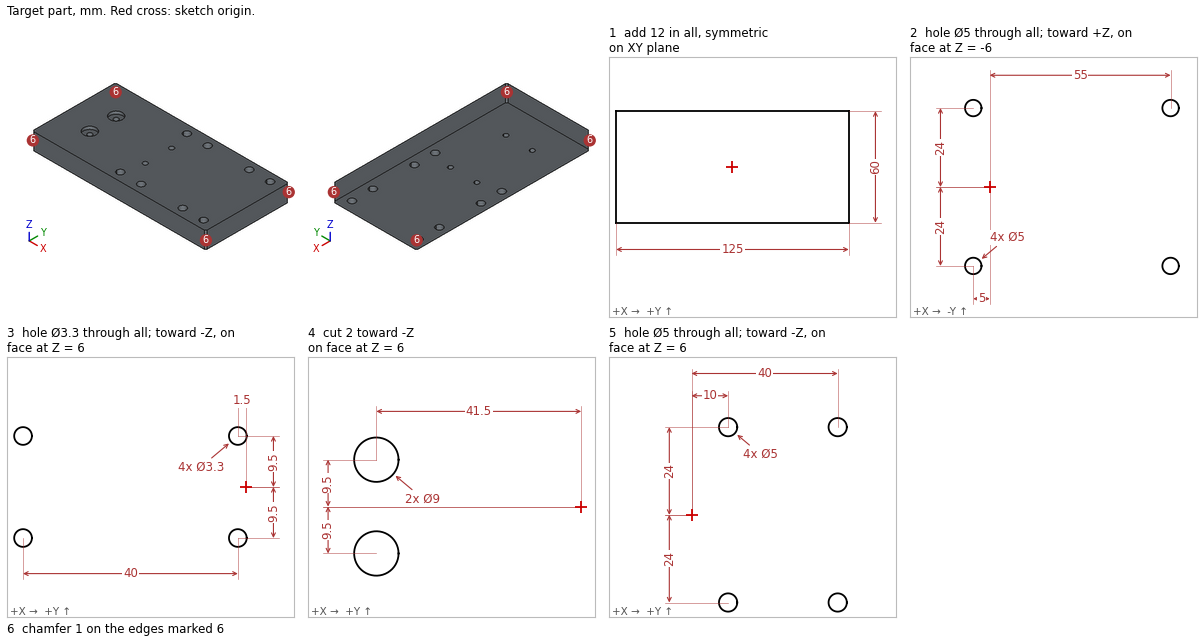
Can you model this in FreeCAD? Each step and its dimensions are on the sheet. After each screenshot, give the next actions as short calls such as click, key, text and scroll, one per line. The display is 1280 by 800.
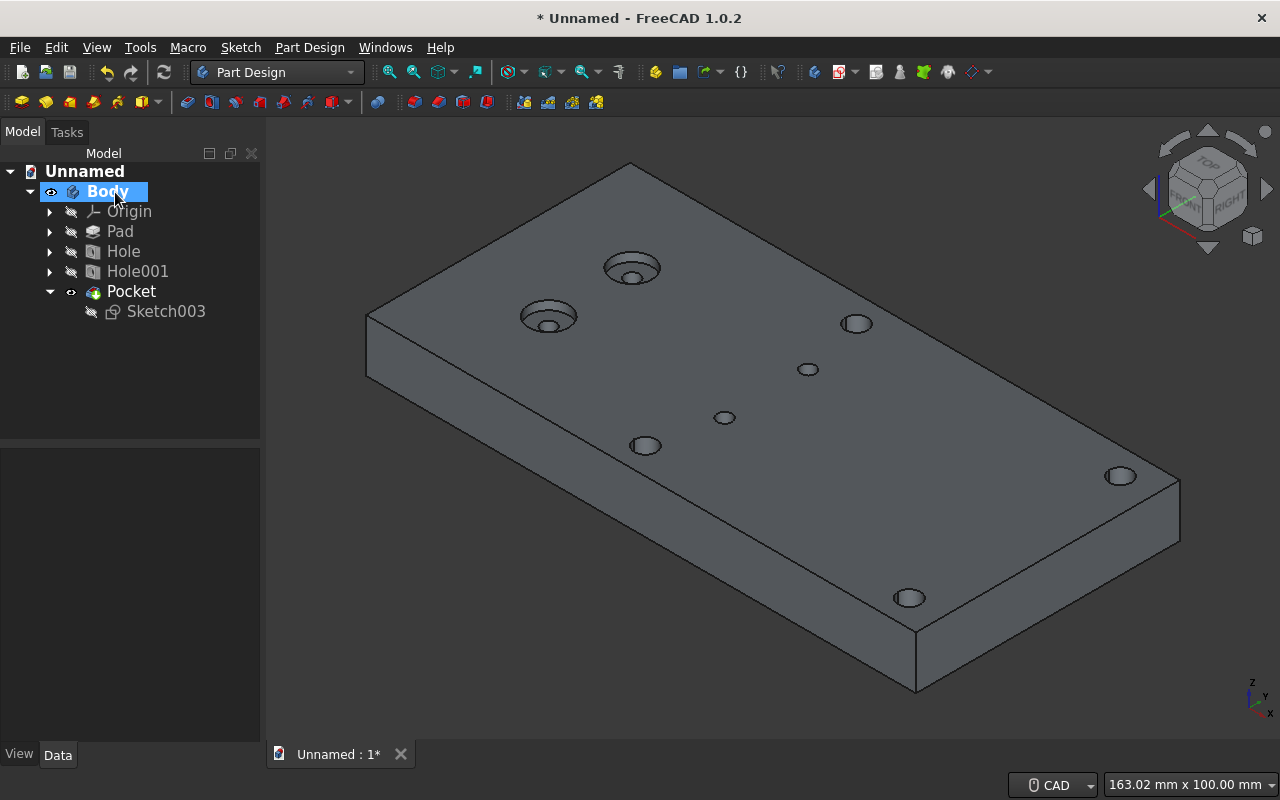
click(930, 487)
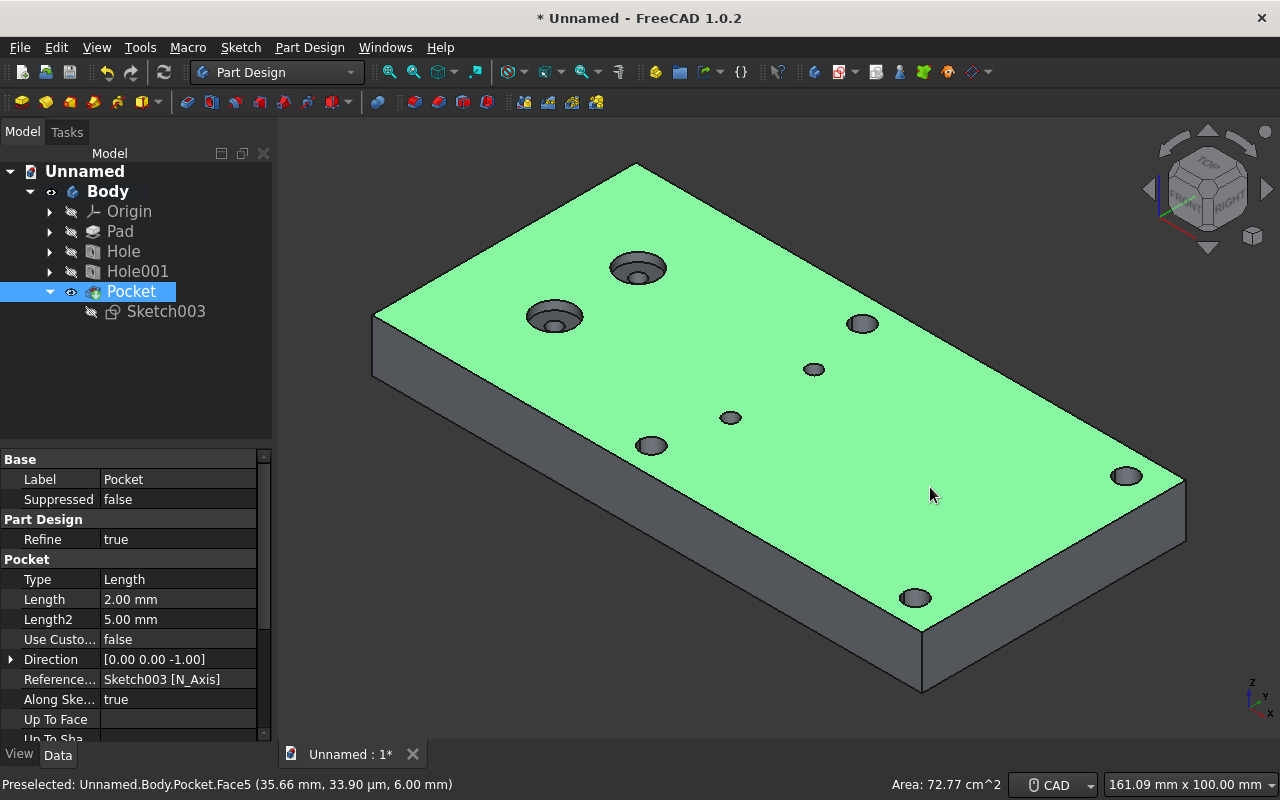
click(840, 72)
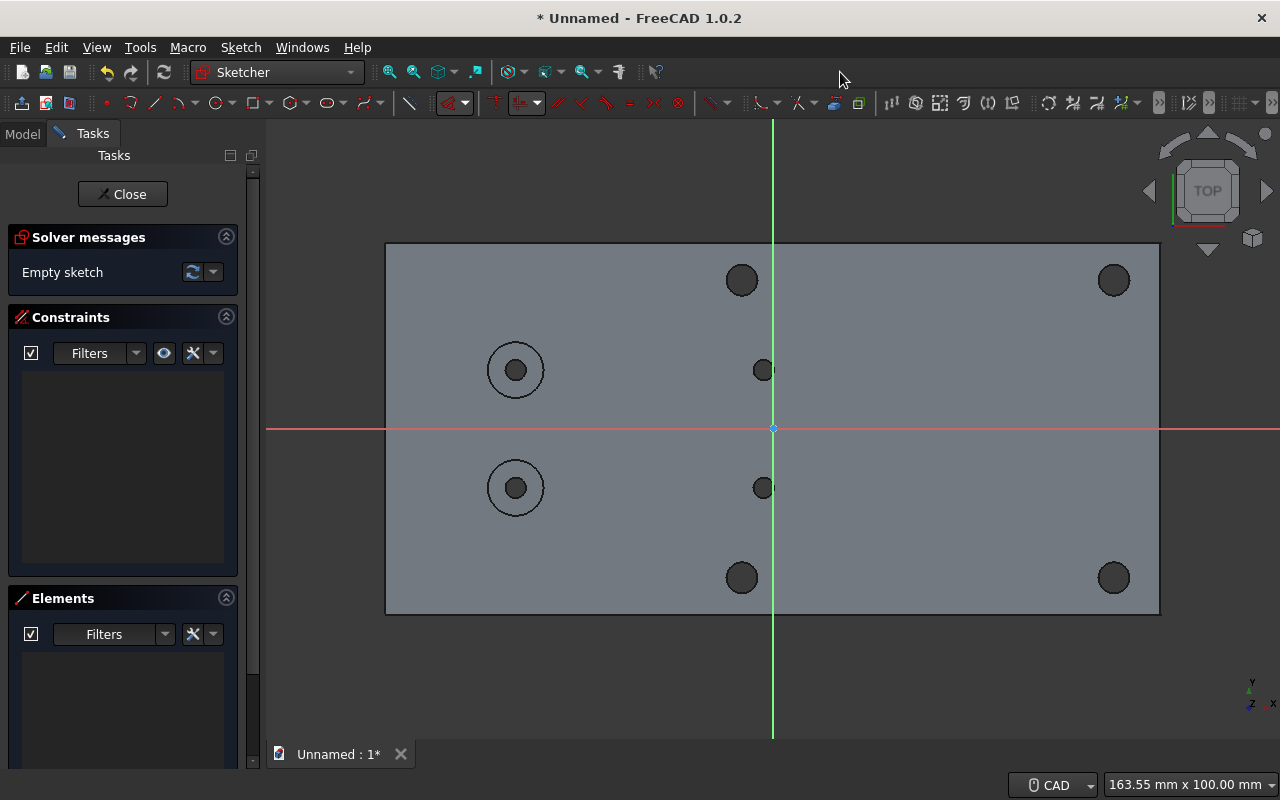
key(g)
key(c)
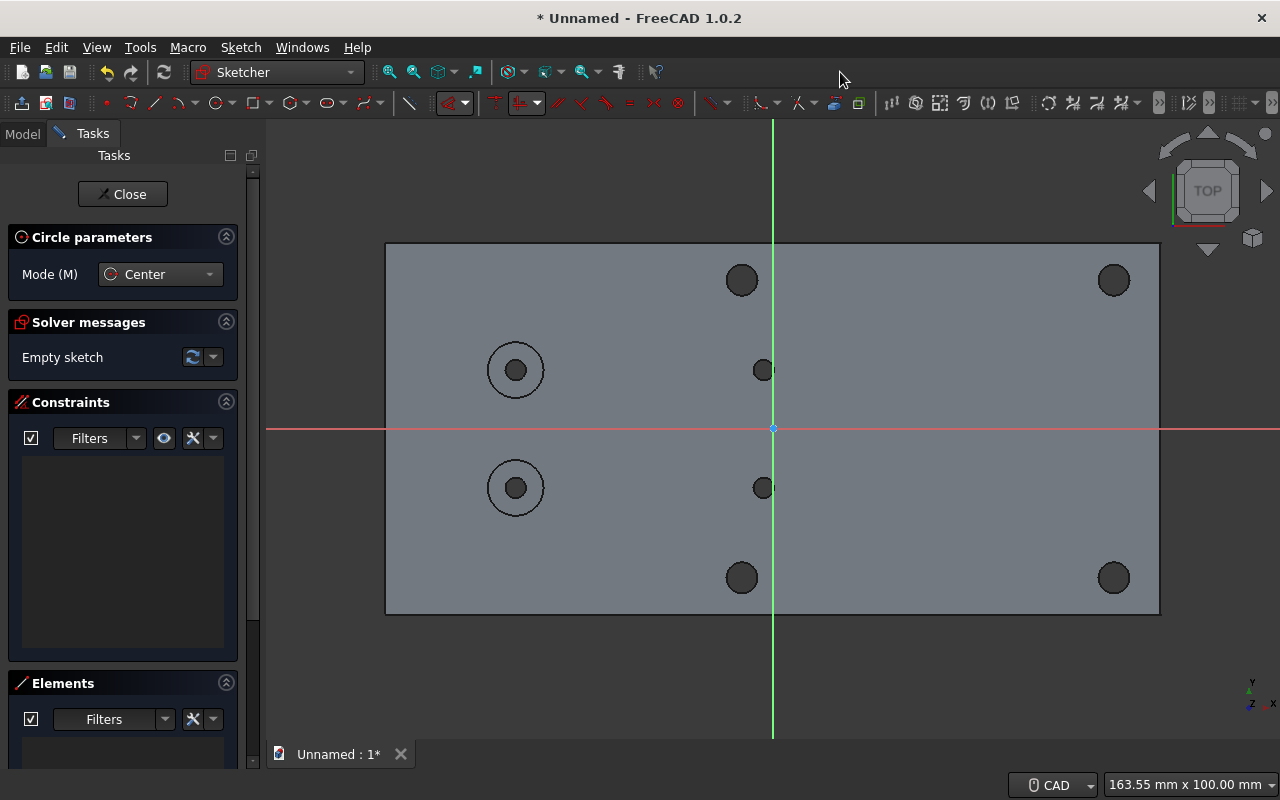
scroll(835, 280, up, 2)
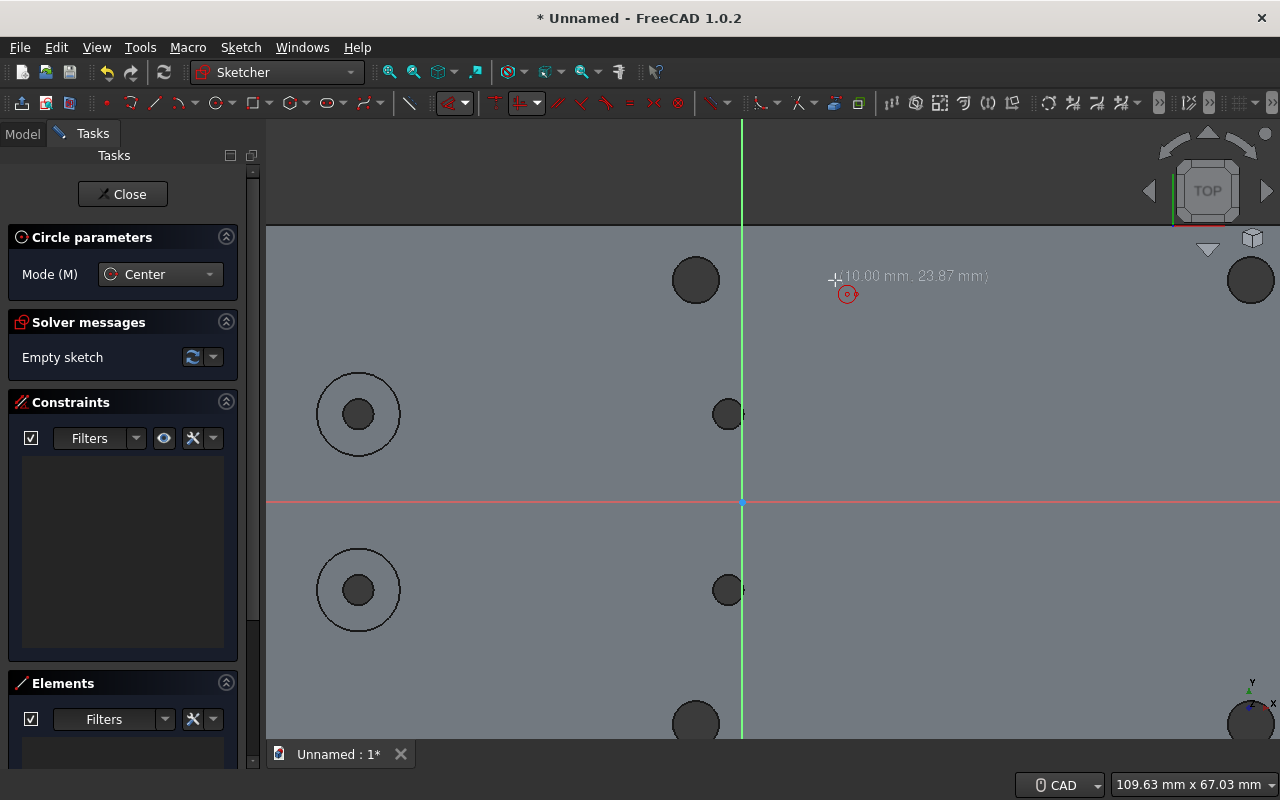
click(835, 280)
click(851, 264)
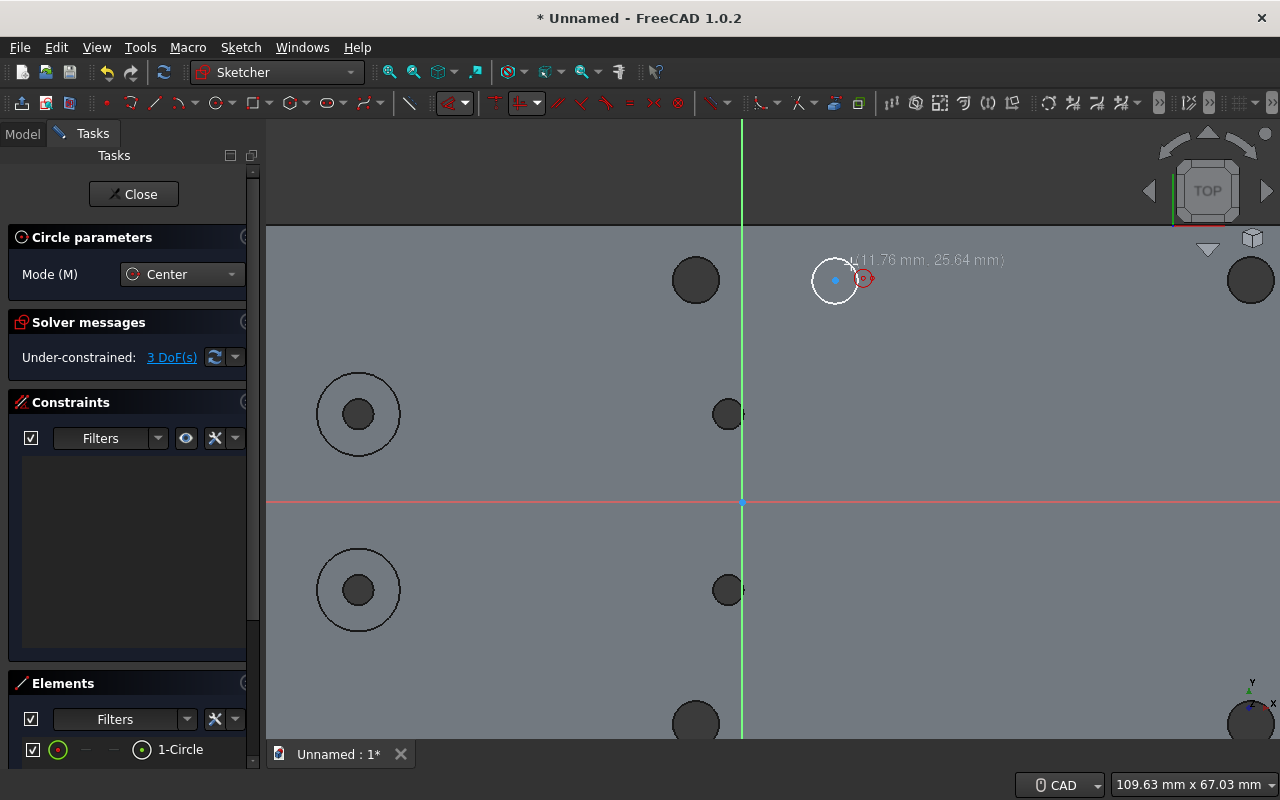
click(1112, 280)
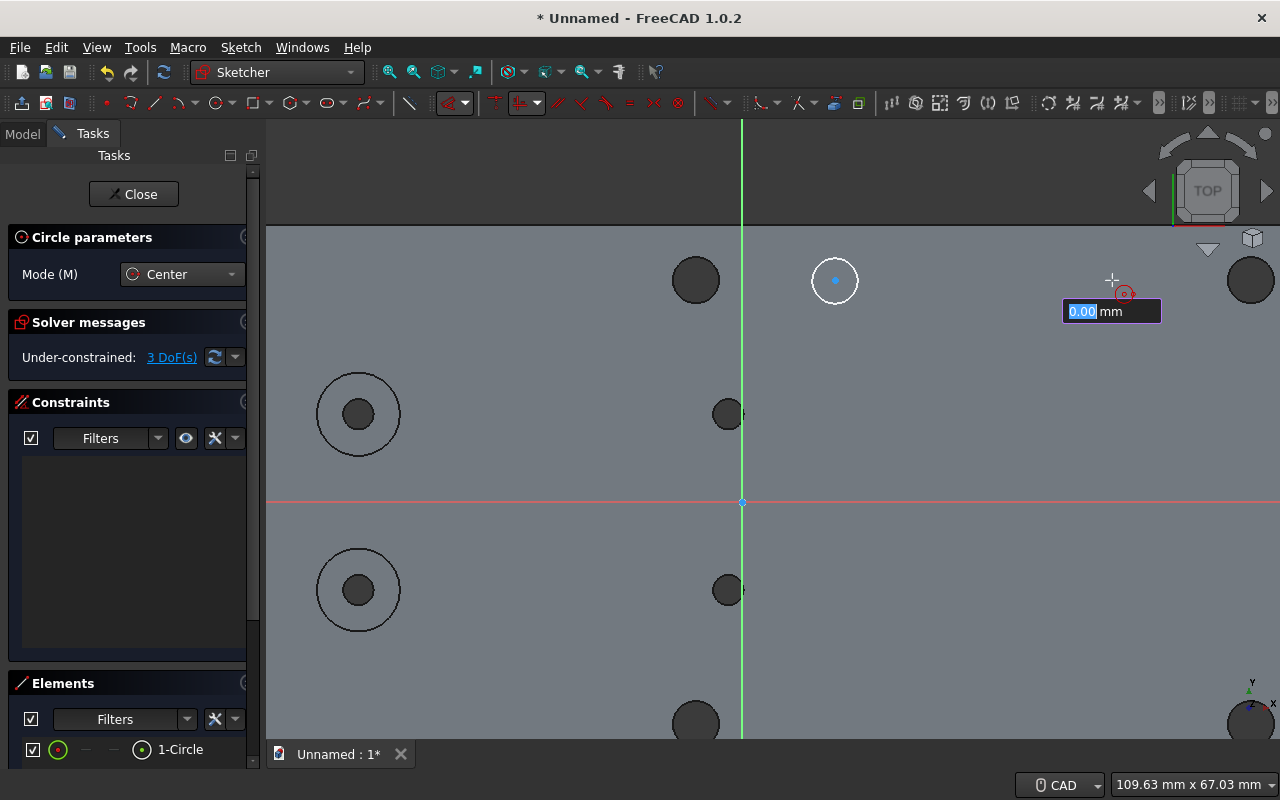
scroll(294, 147, down, 1)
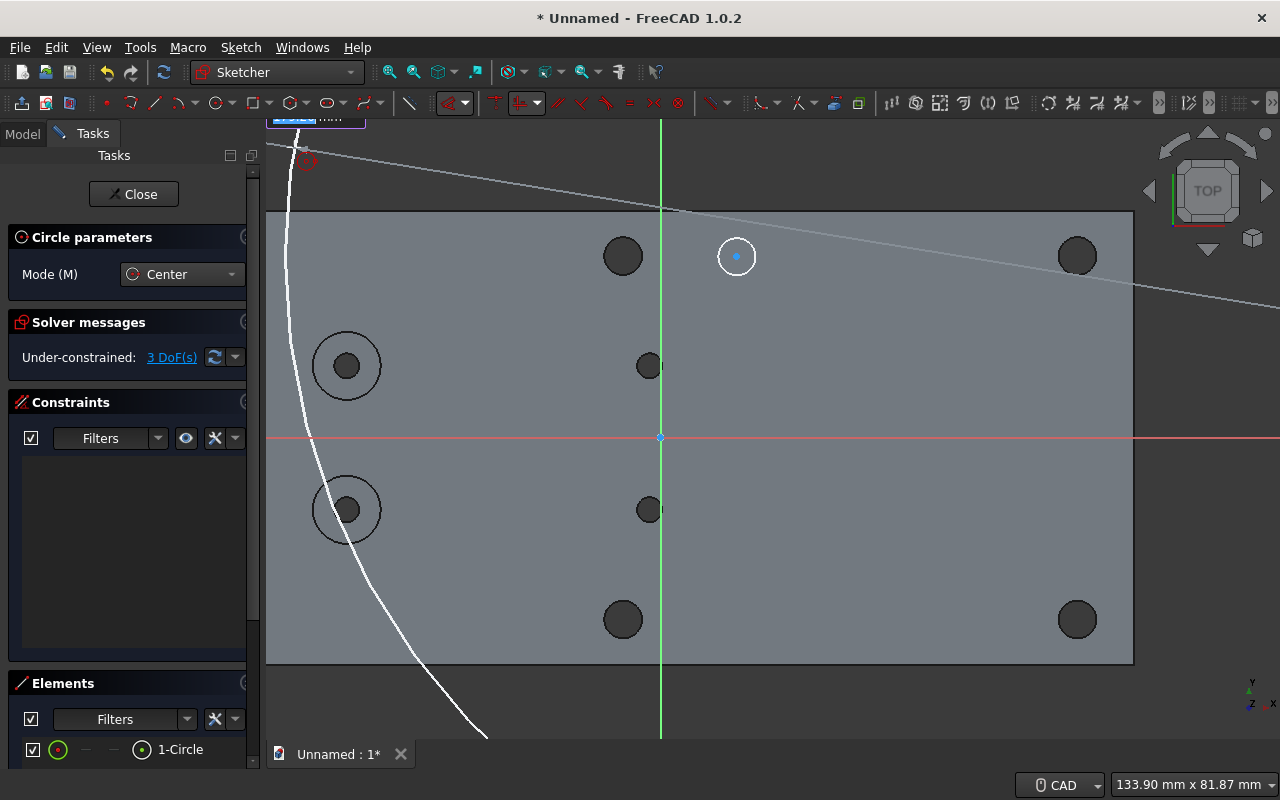
click(977, 243)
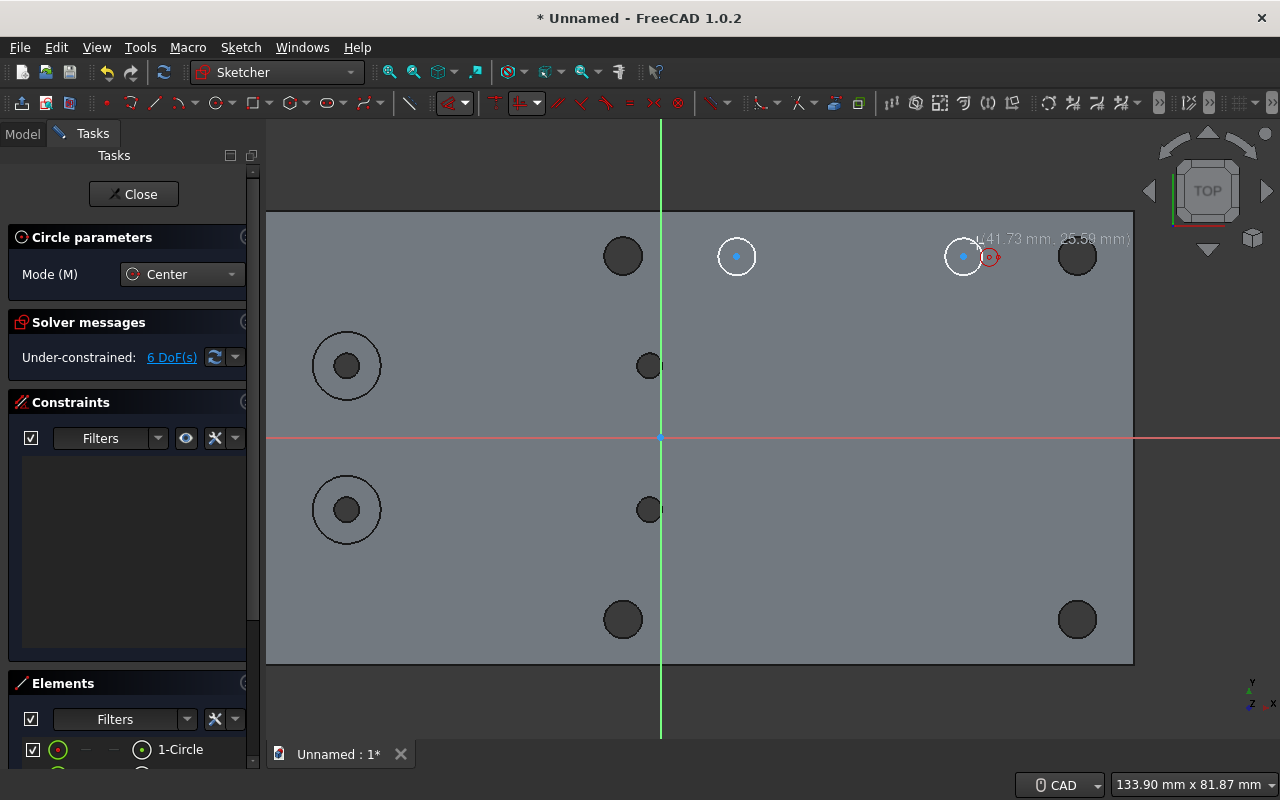
click(737, 620)
click(750, 606)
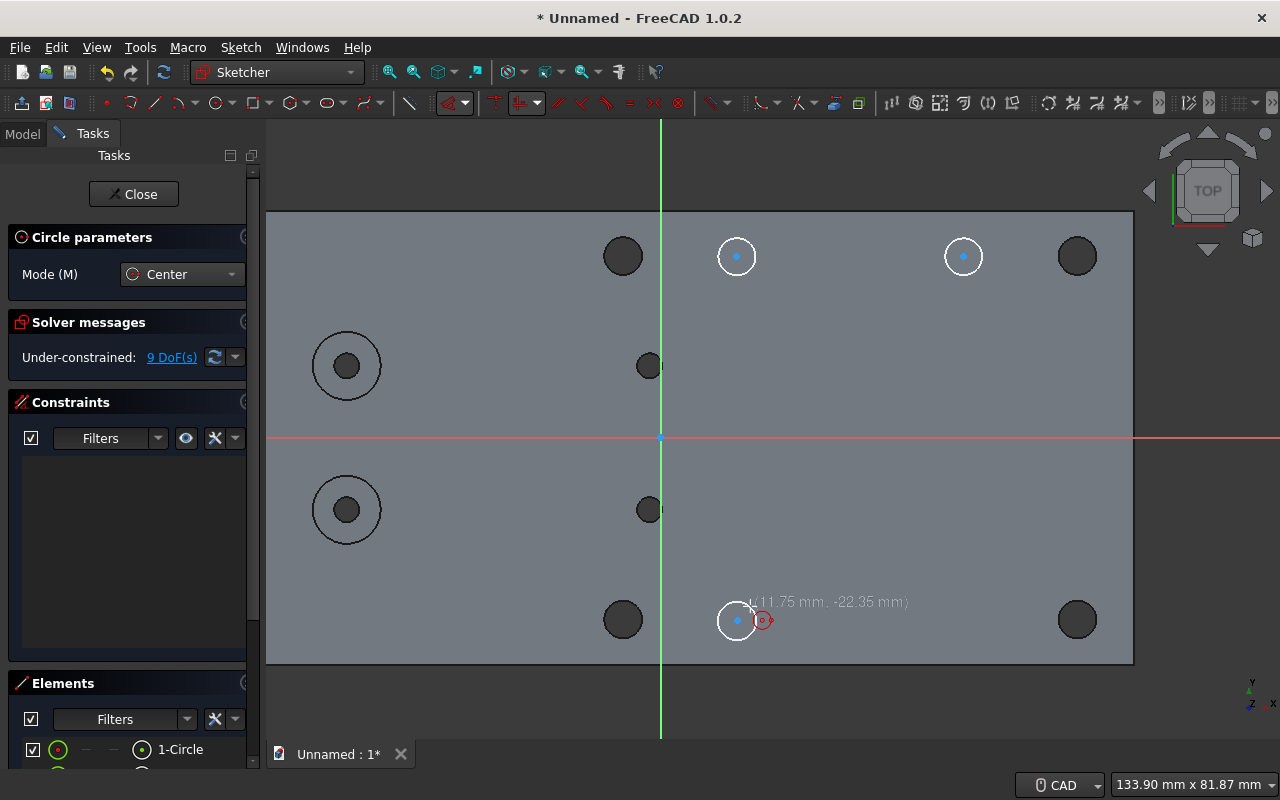
click(964, 620)
click(977, 606)
key(Escape)